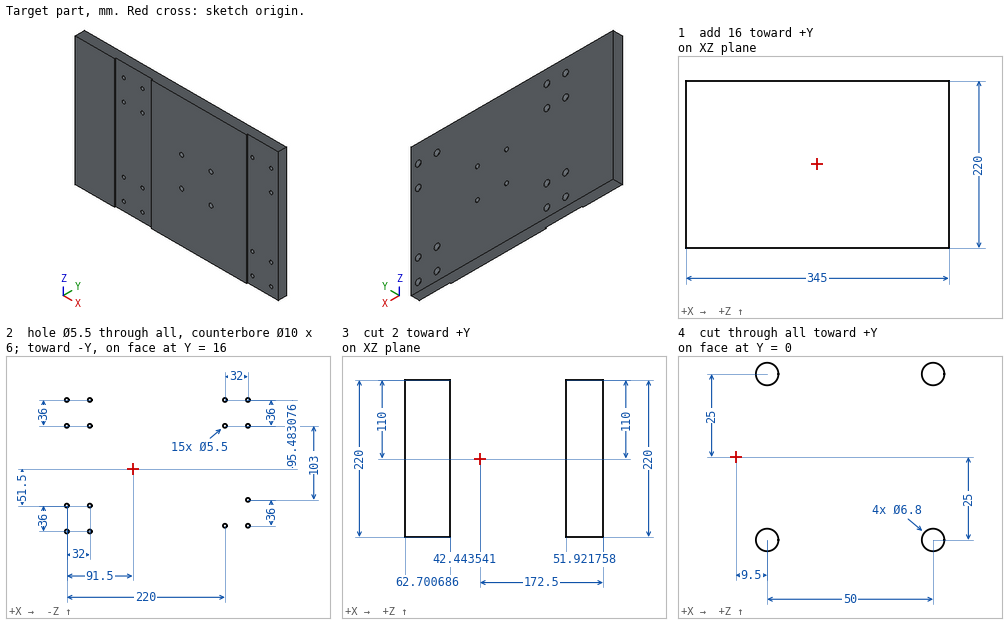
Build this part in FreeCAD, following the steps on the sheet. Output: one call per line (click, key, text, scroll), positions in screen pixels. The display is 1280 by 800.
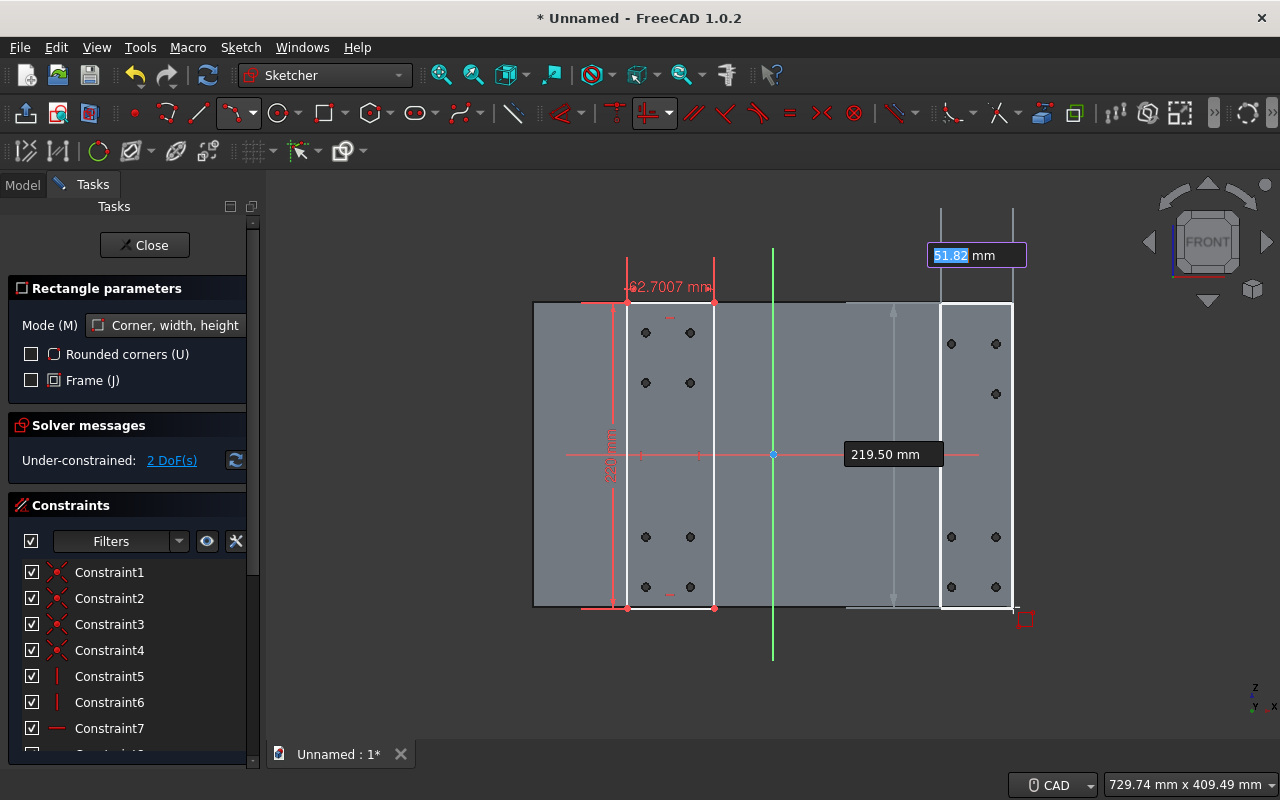
text(51.921758)
key(Tab)
text(220)
key(Return)
key(Escape)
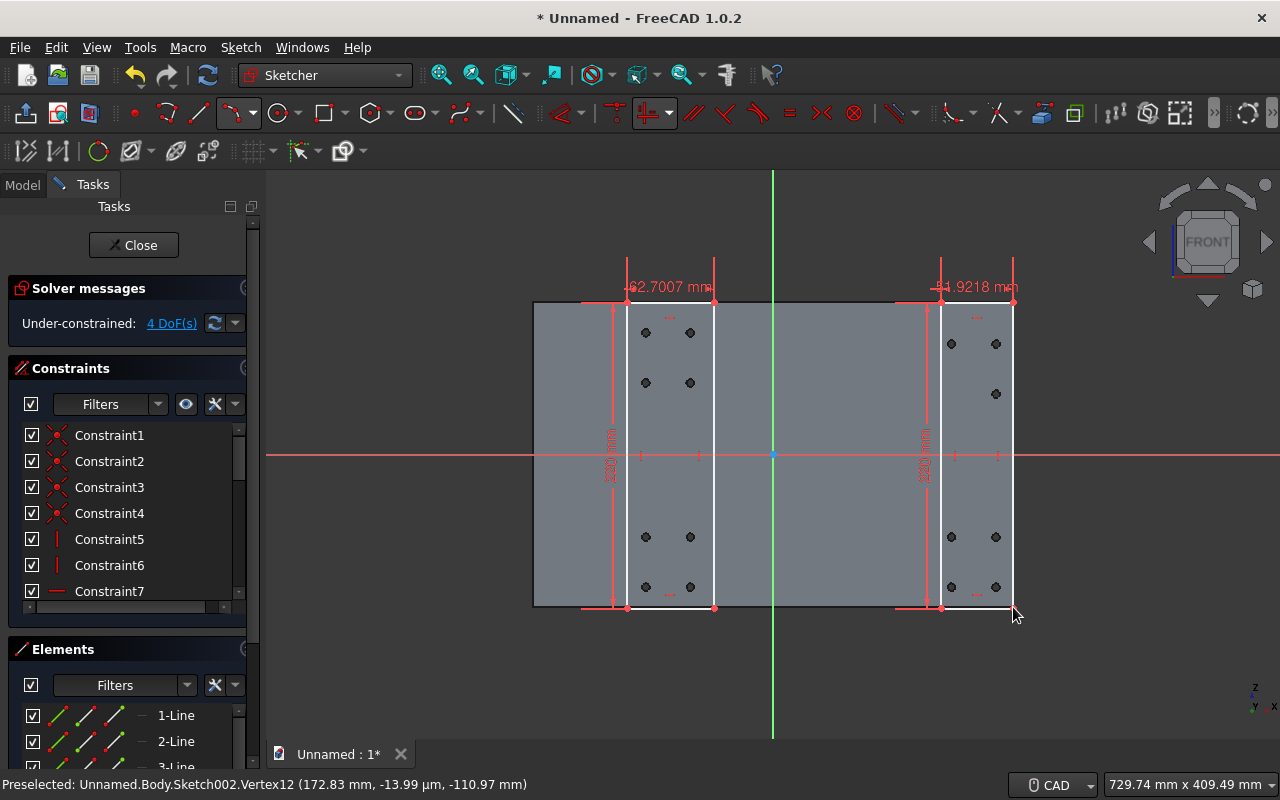
click(560, 114)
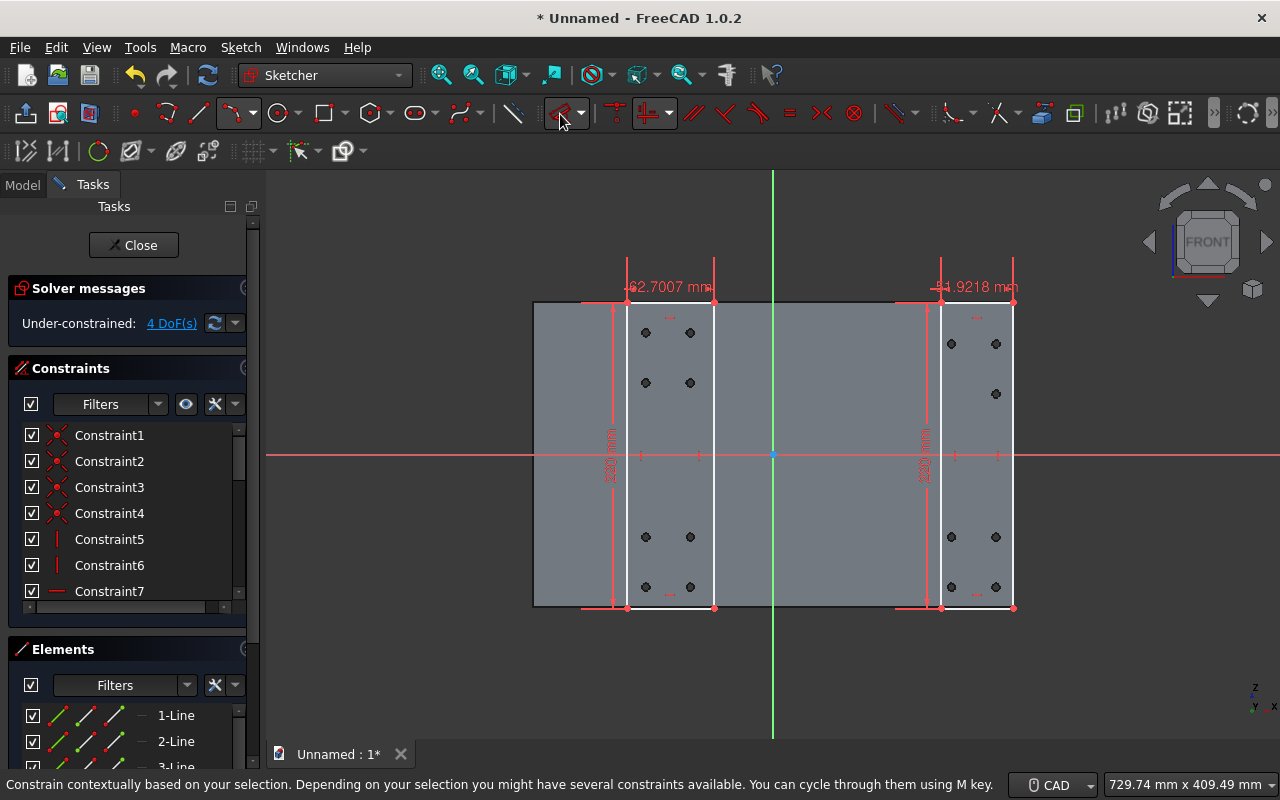
click(627, 303)
click(593, 379)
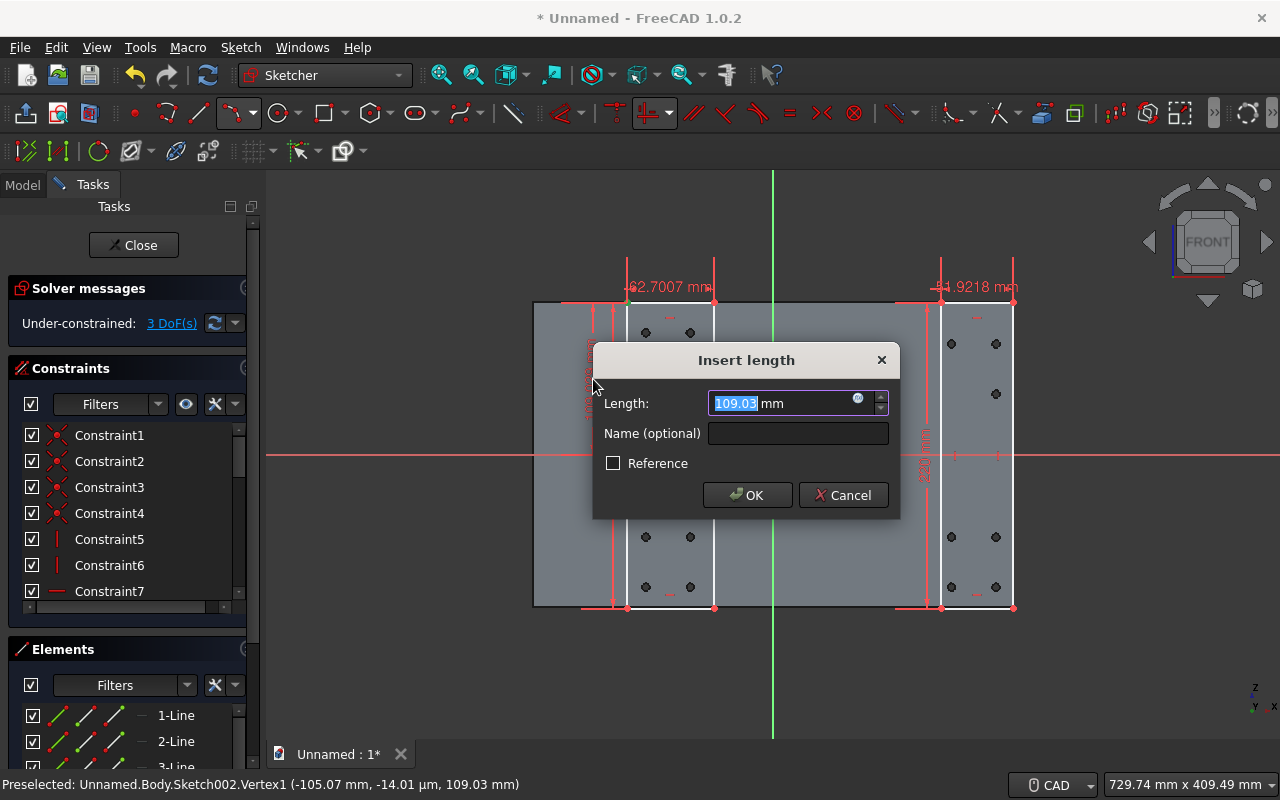
text(110)
key(Return)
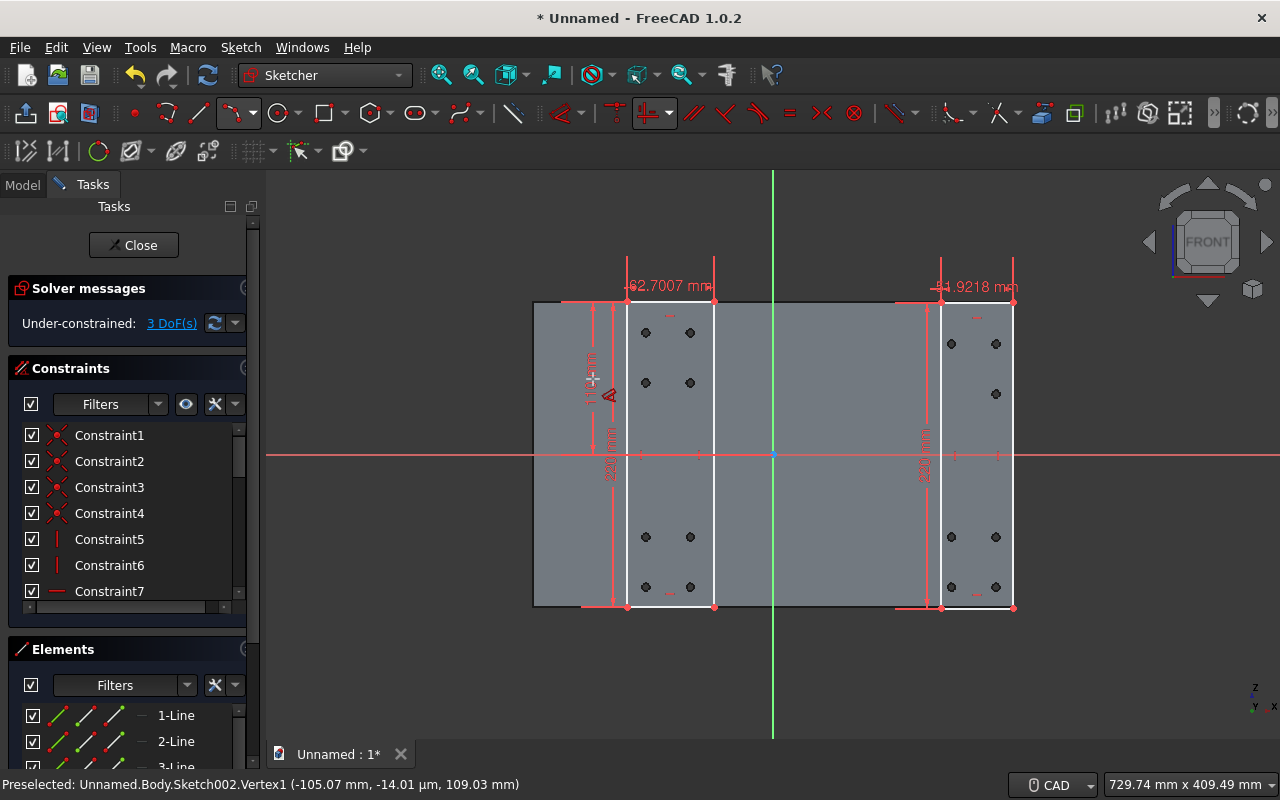
click(941, 303)
click(975, 379)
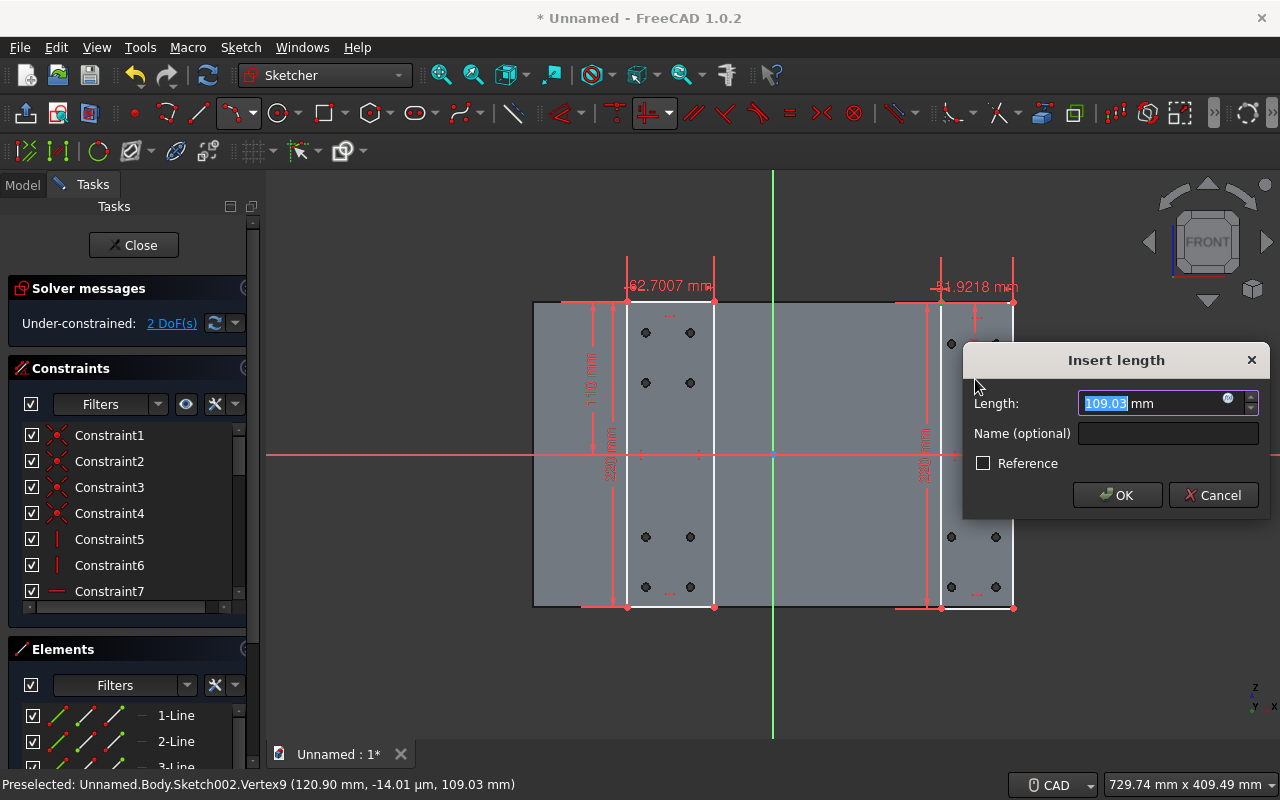
text(110)
key(Return)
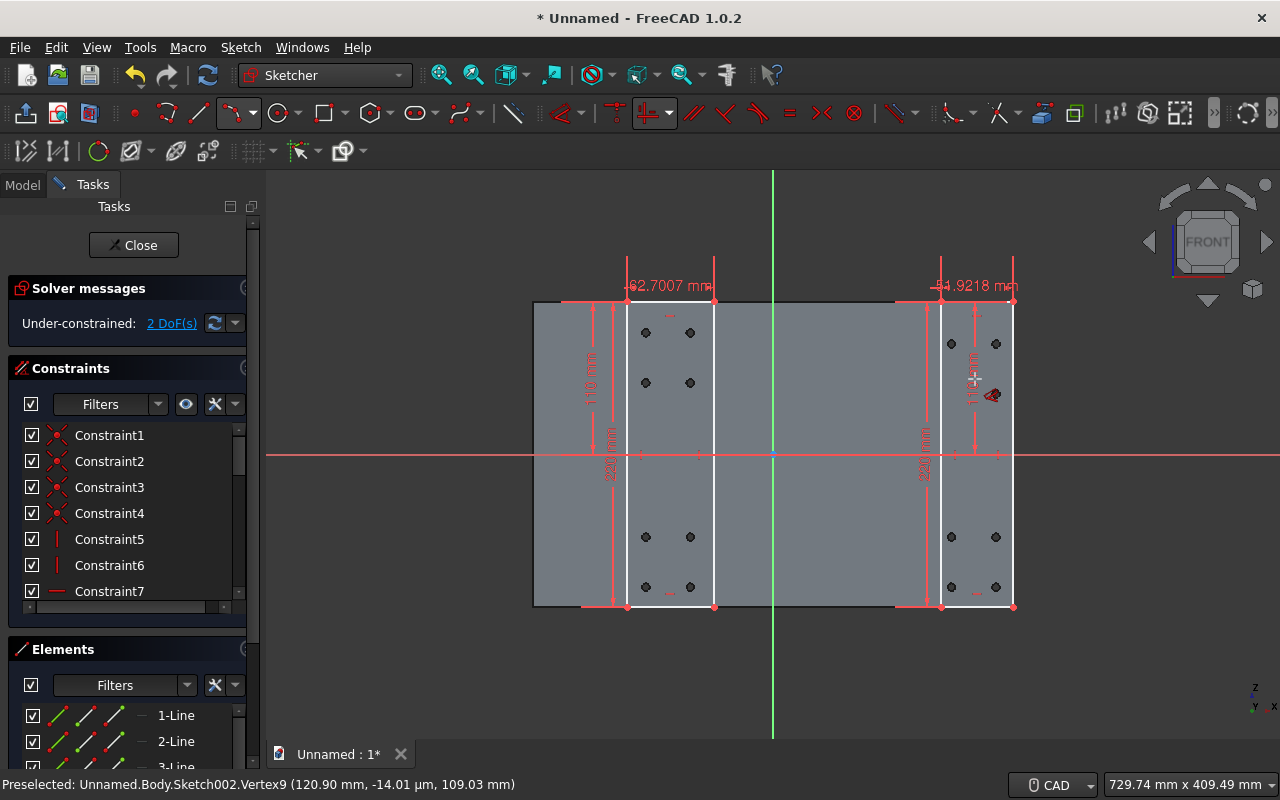
click(1013, 607)
click(893, 641)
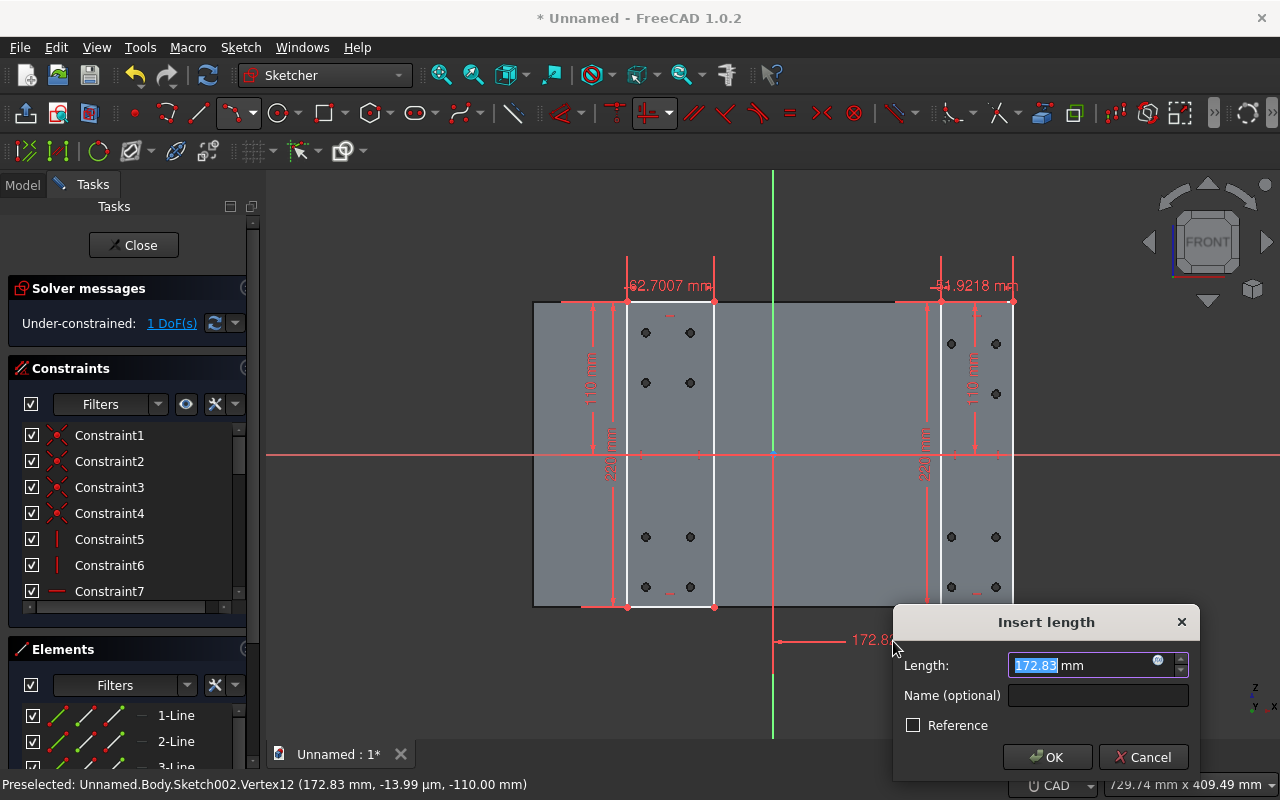
text(172.5)
key(Return)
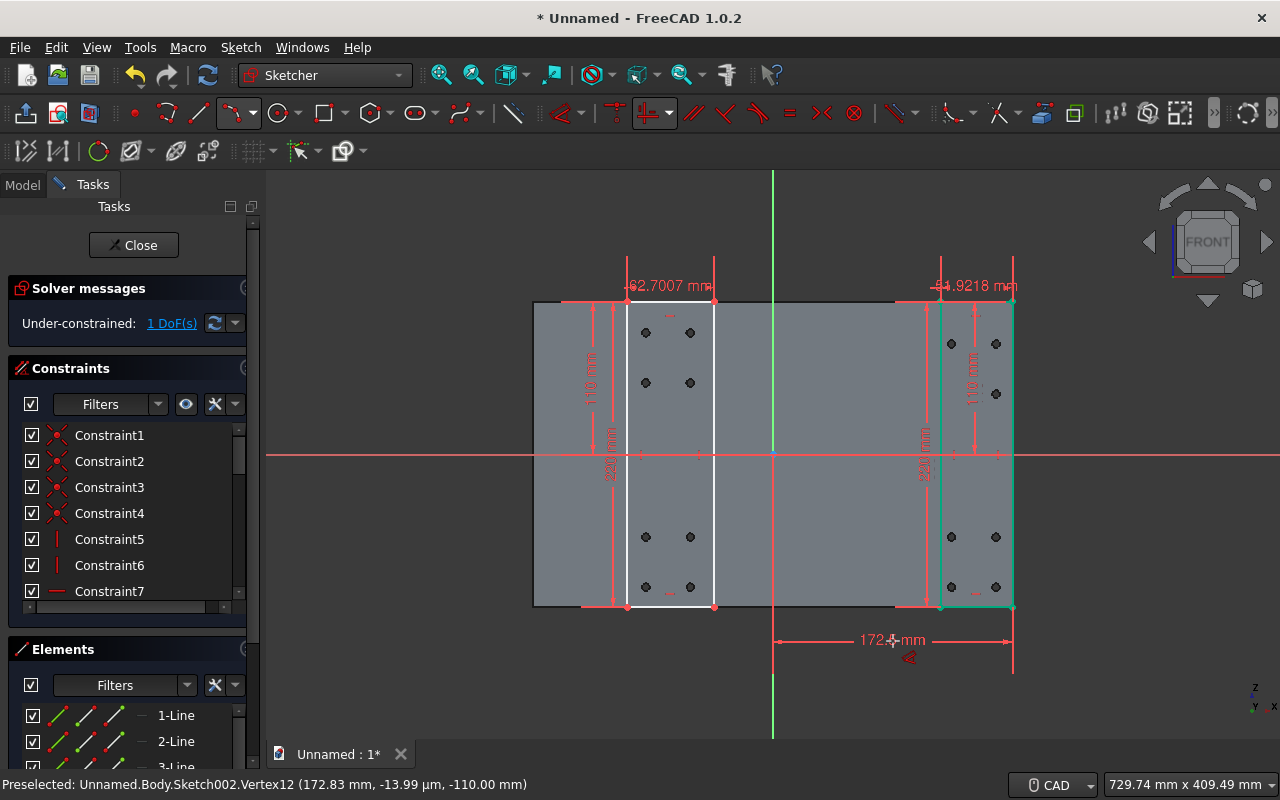
click(714, 607)
click(744, 641)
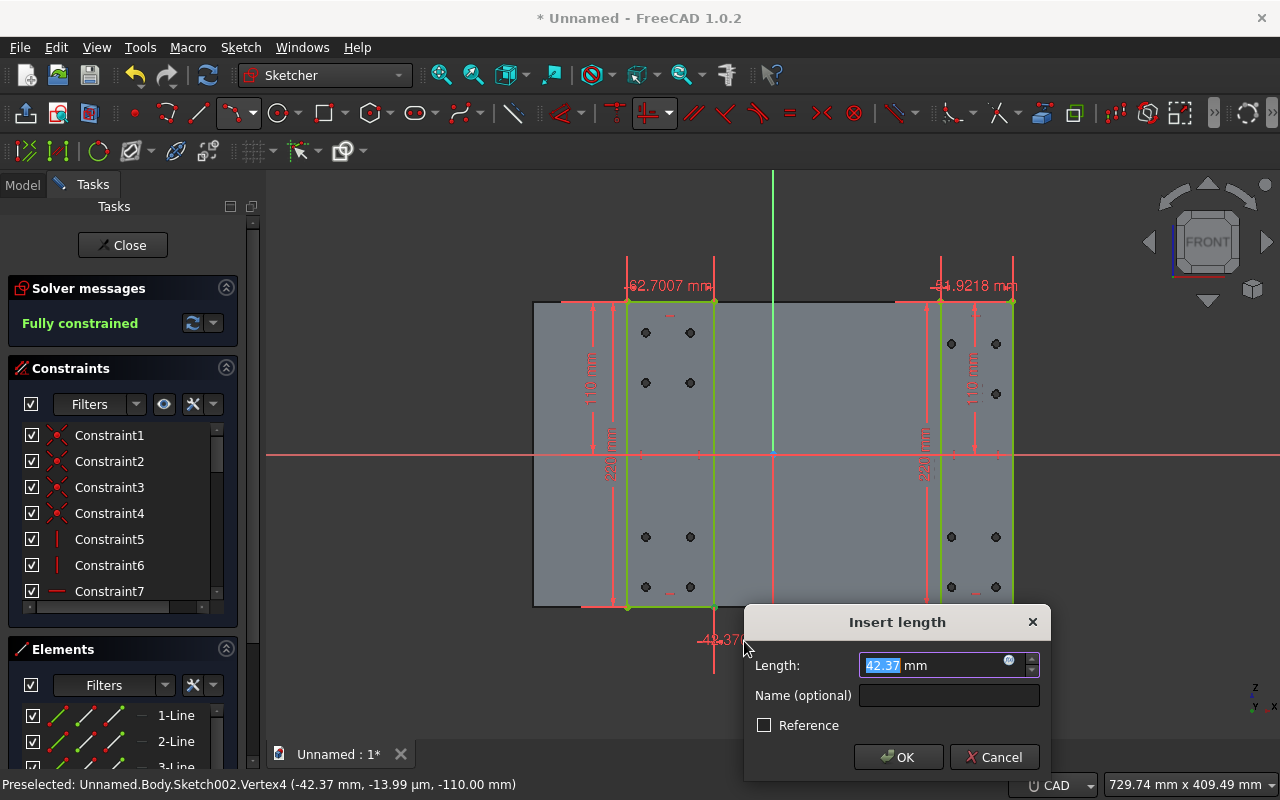
text(42.443541)
key(Return)
key(Escape)